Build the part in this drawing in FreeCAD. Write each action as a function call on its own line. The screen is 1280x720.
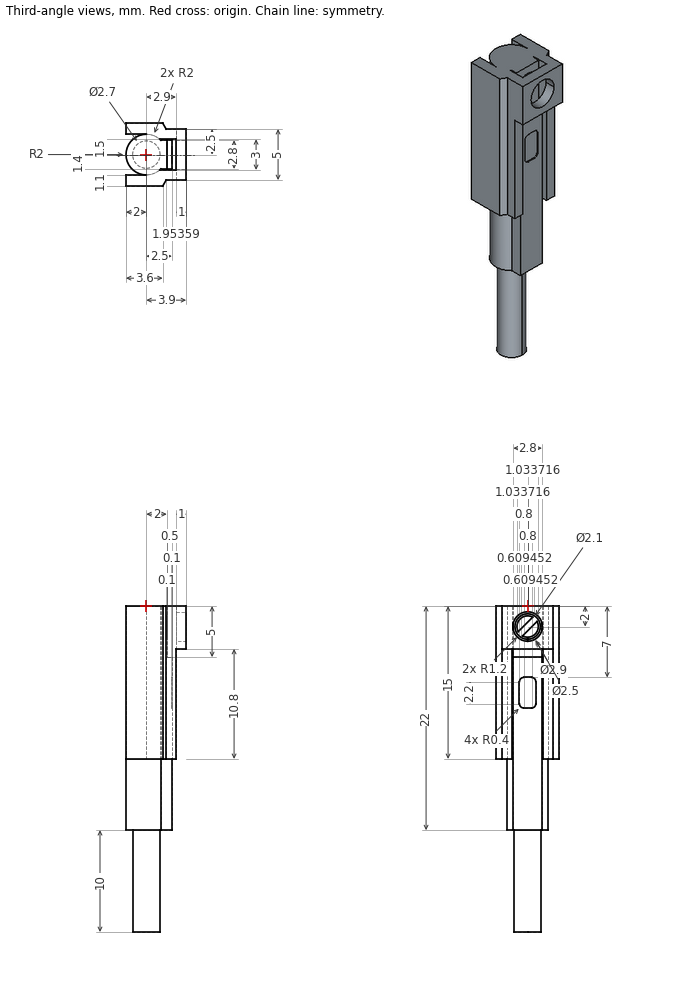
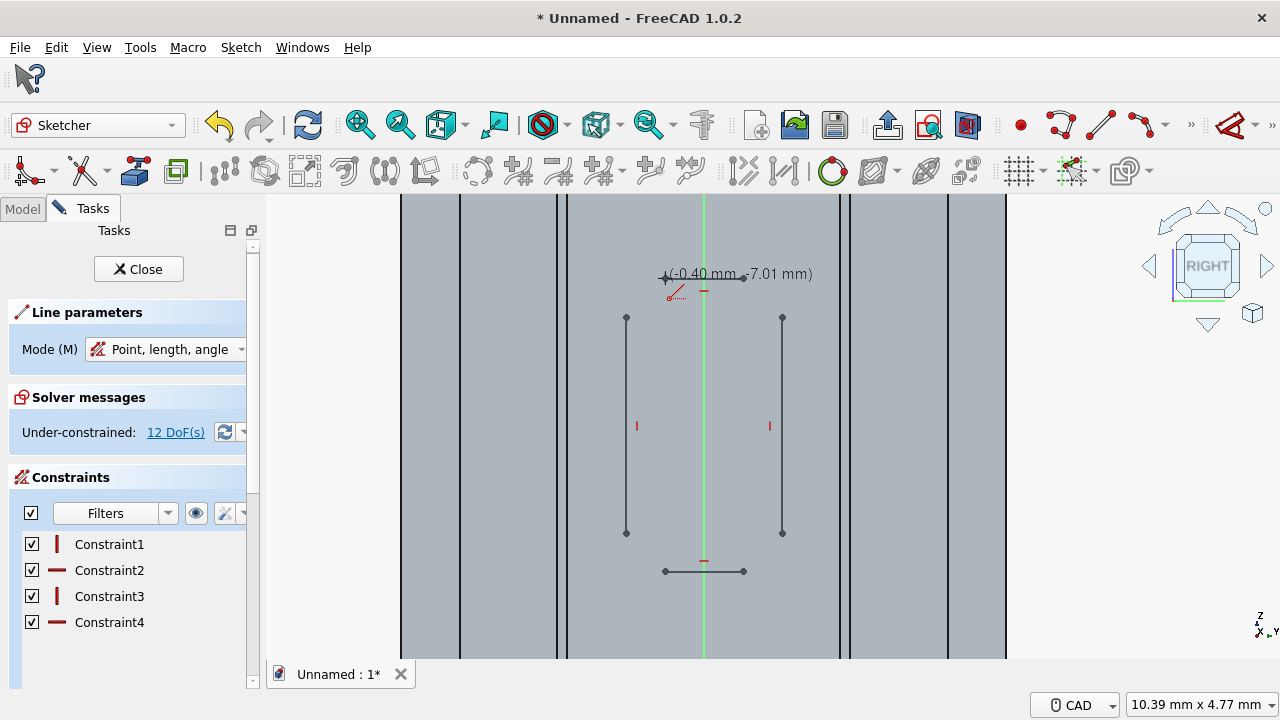
click(1142, 126)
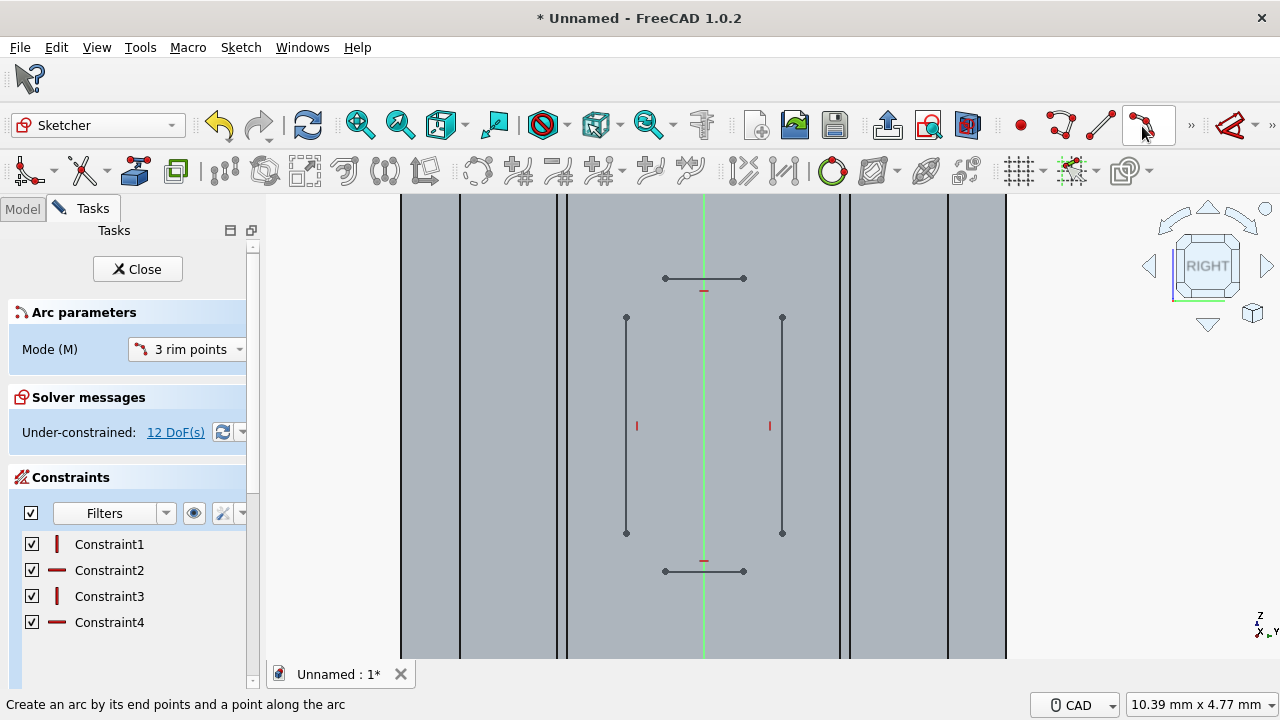
click(626, 533)
click(665, 572)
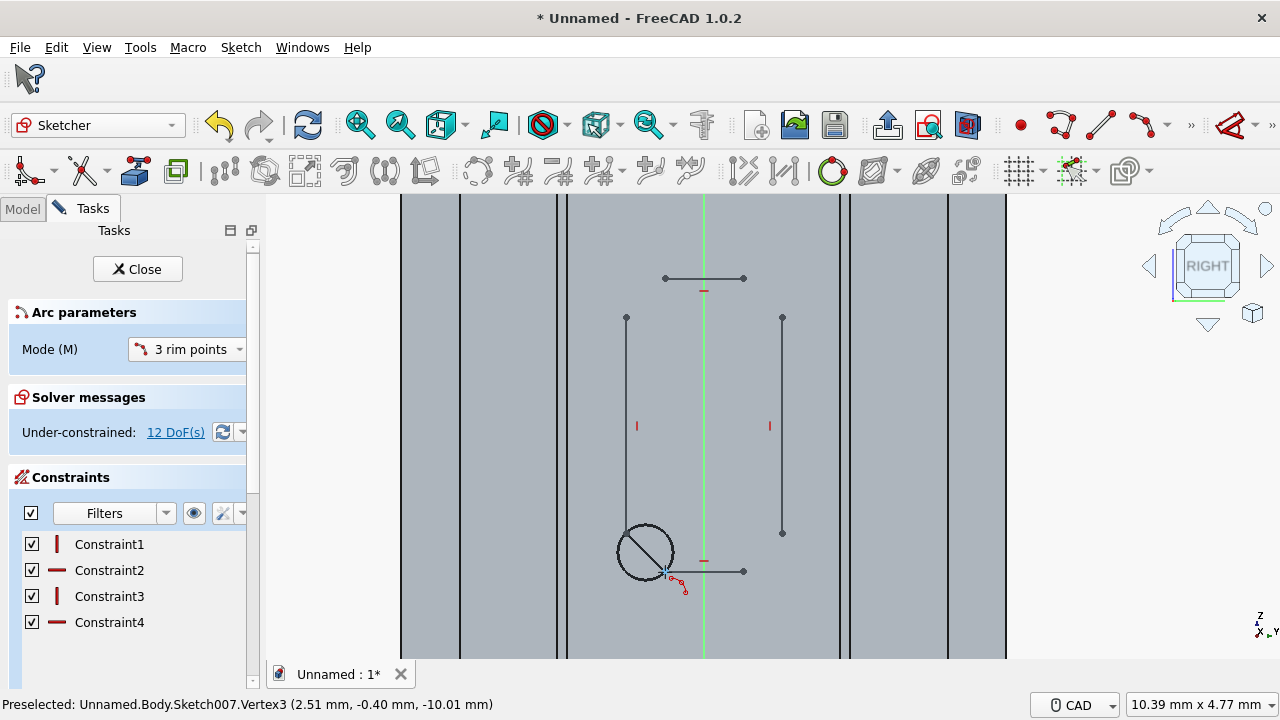
scroll(637, 559, up, 2)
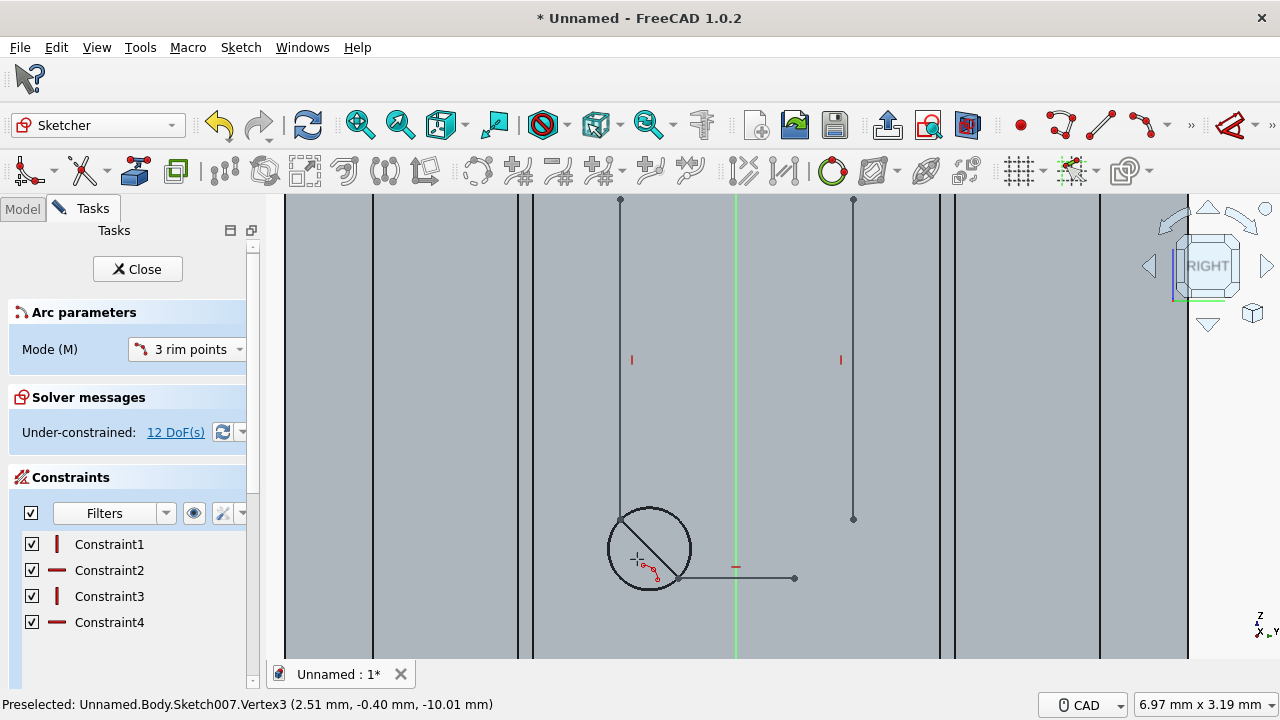
click(637, 559)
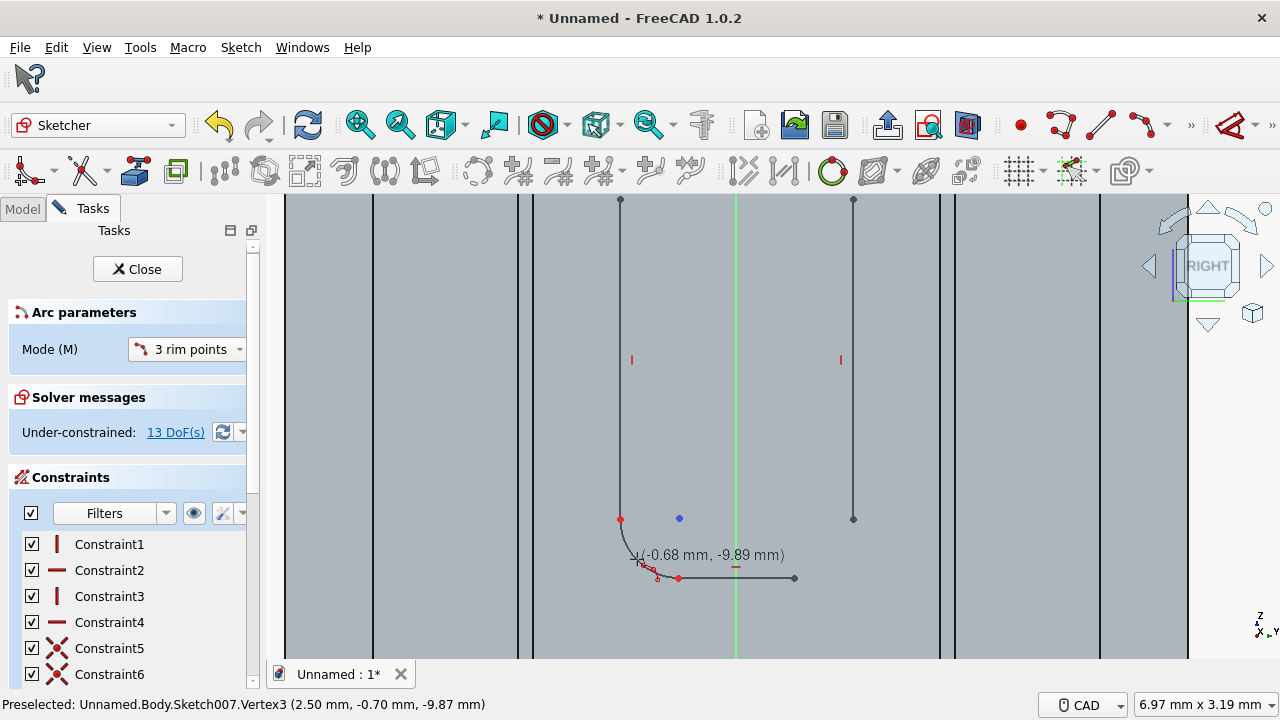
click(795, 578)
click(853, 520)
click(836, 559)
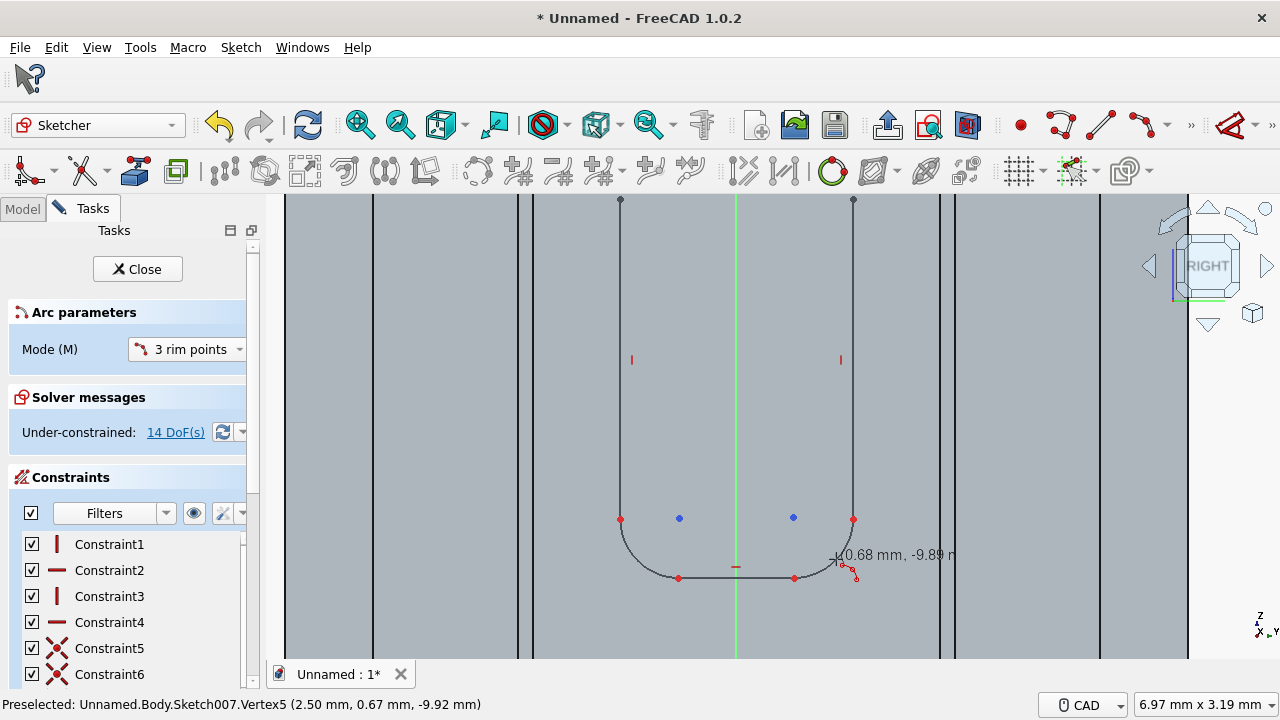
scroll(640, 567, down, 2)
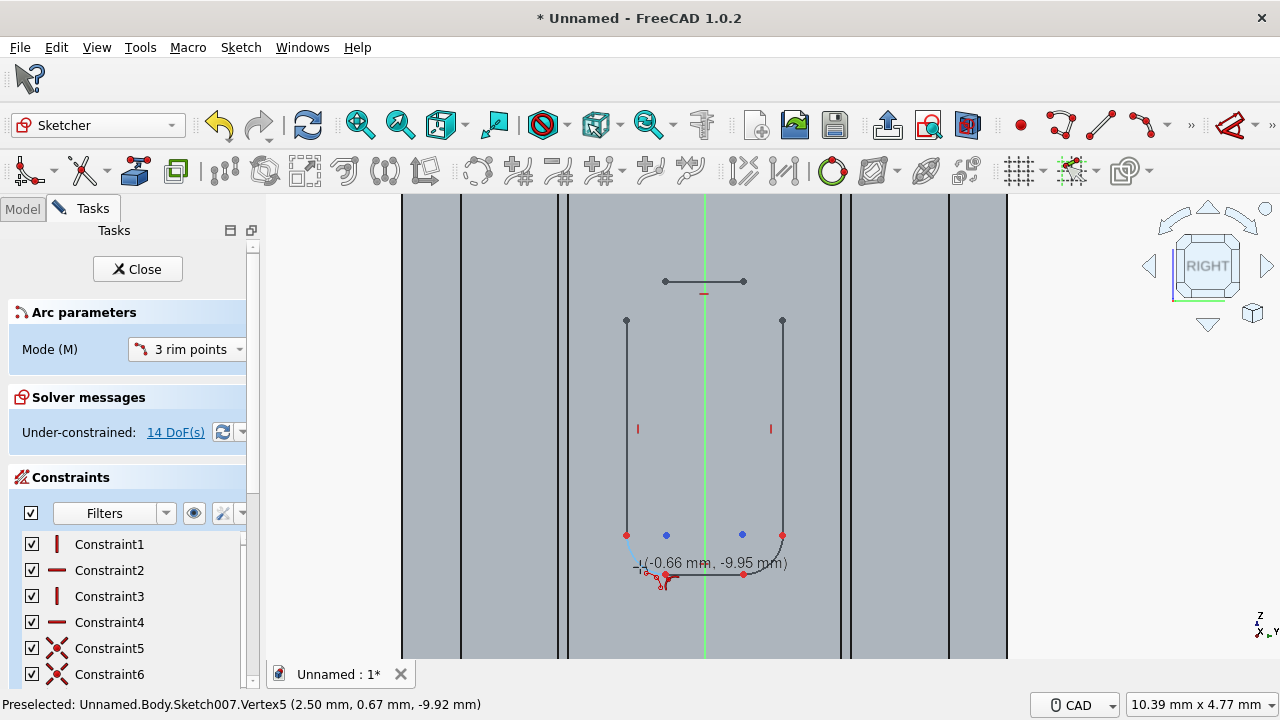
click(783, 321)
click(744, 282)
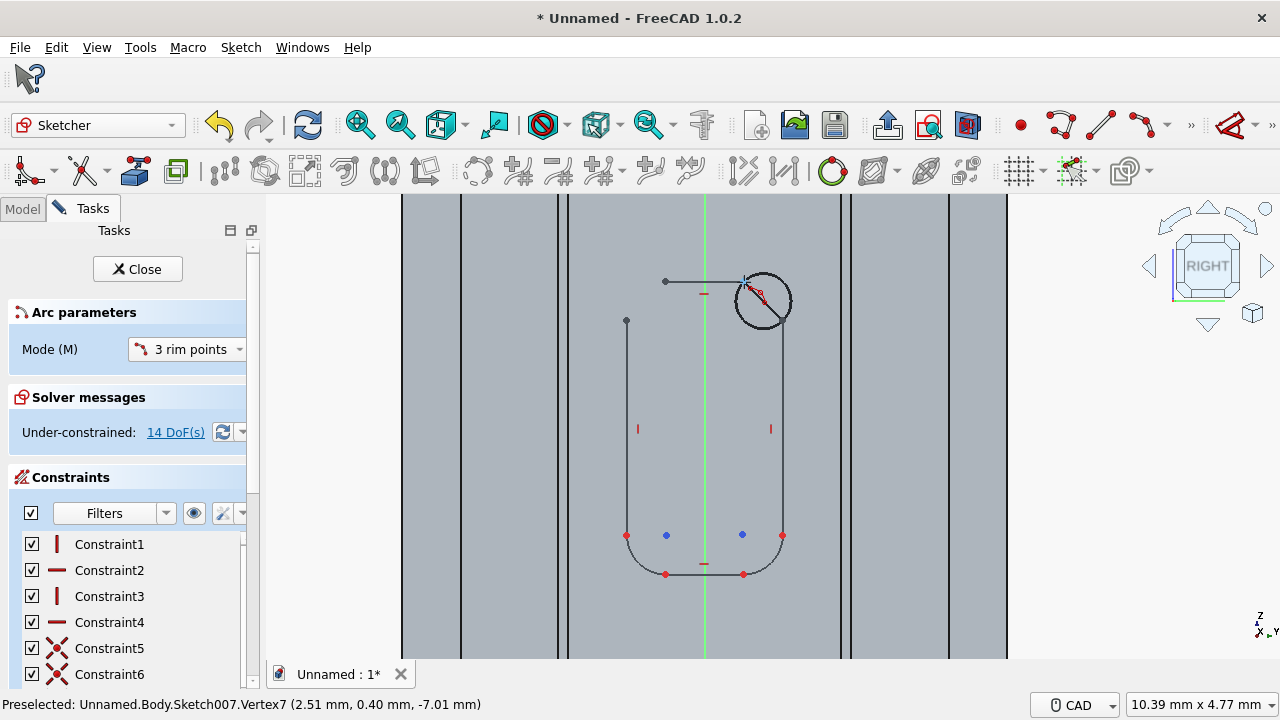
scroll(771, 292, up, 2)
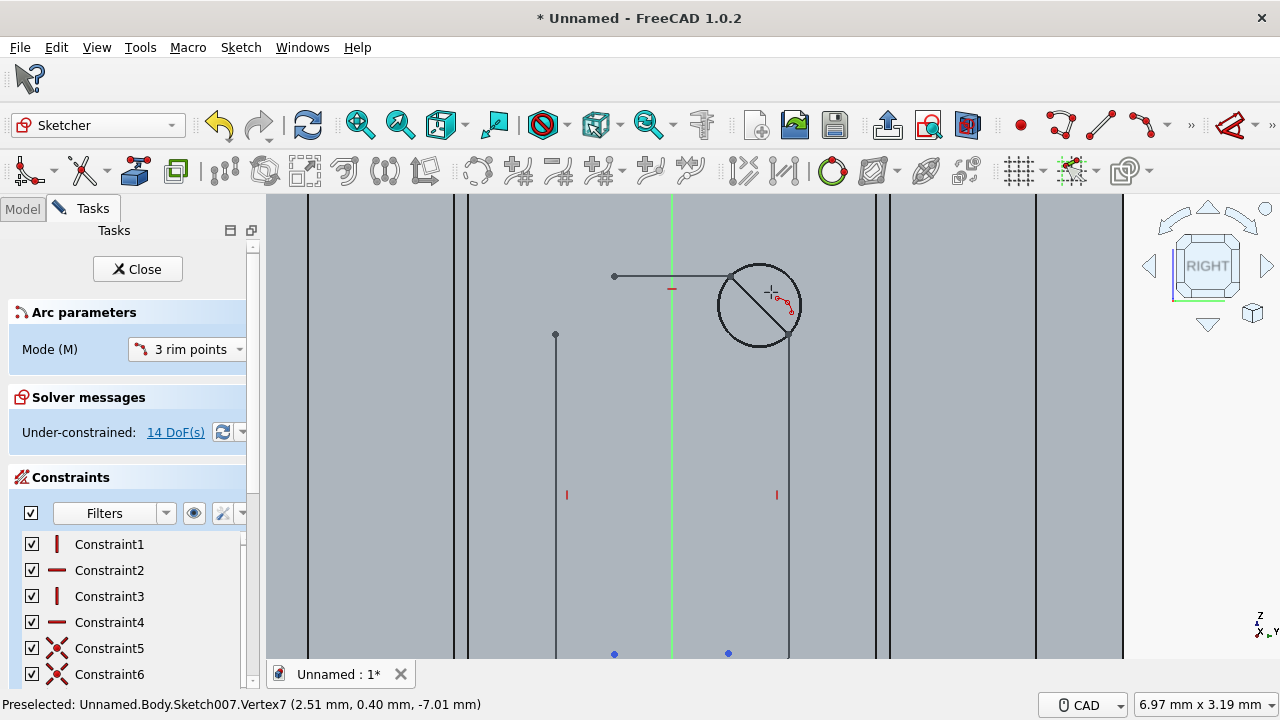
click(771, 292)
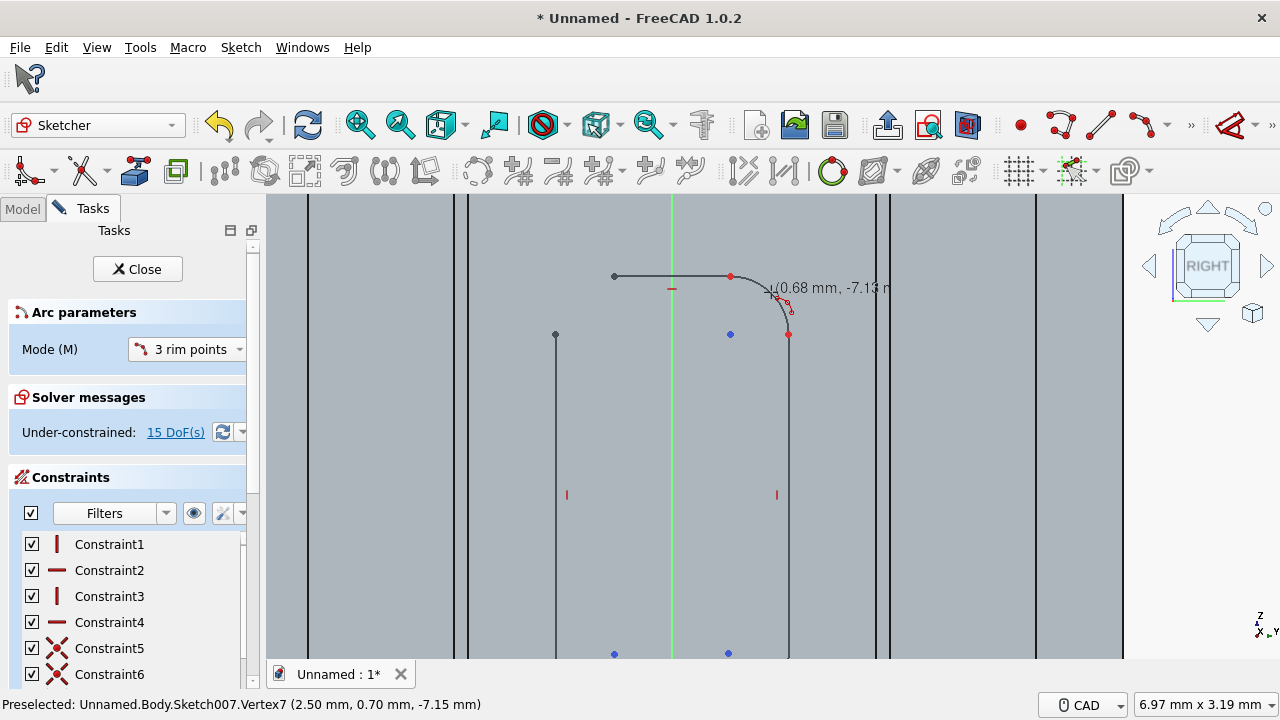
click(614, 276)
click(556, 335)
click(573, 292)
key(Escape)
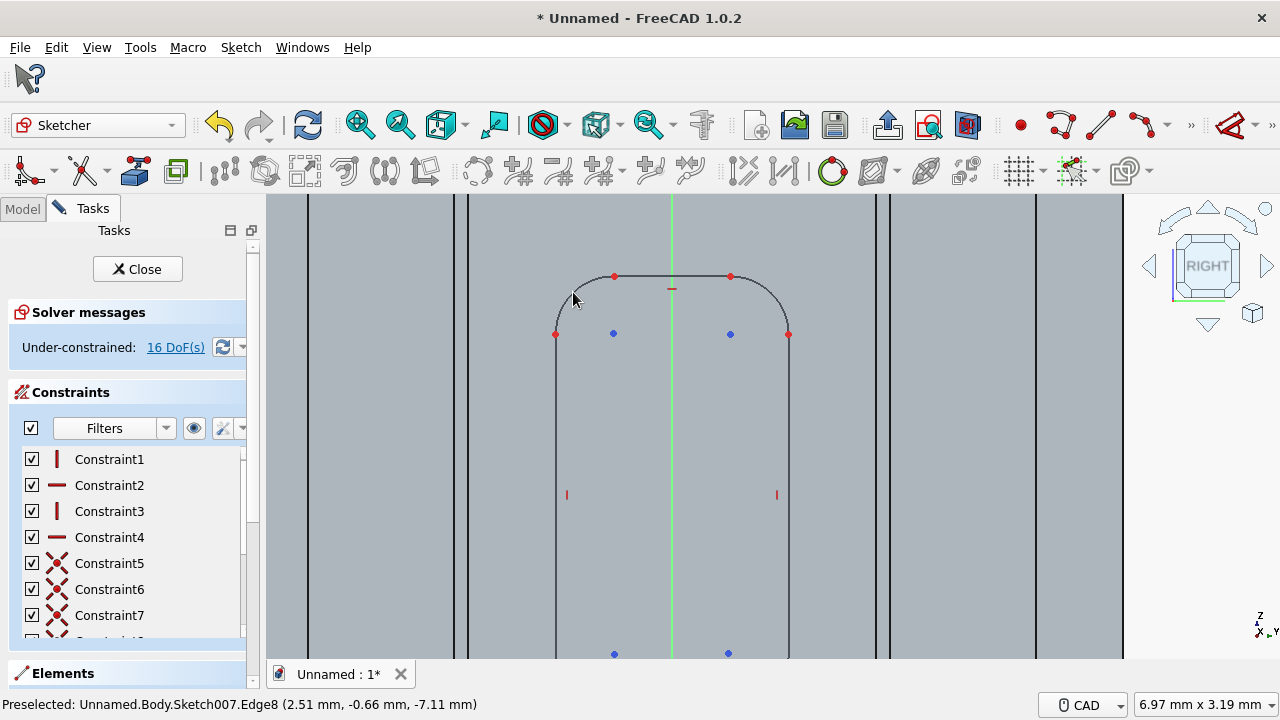
click(556, 431)